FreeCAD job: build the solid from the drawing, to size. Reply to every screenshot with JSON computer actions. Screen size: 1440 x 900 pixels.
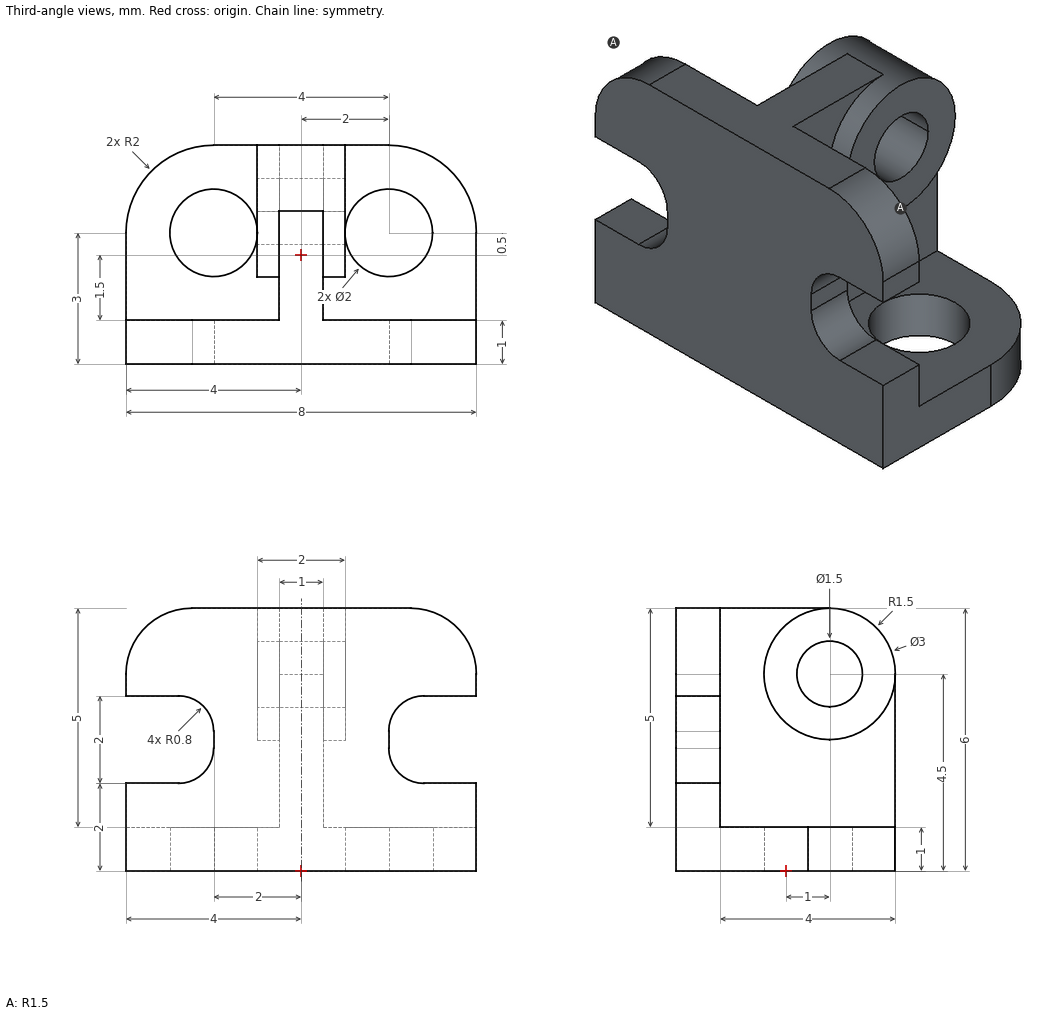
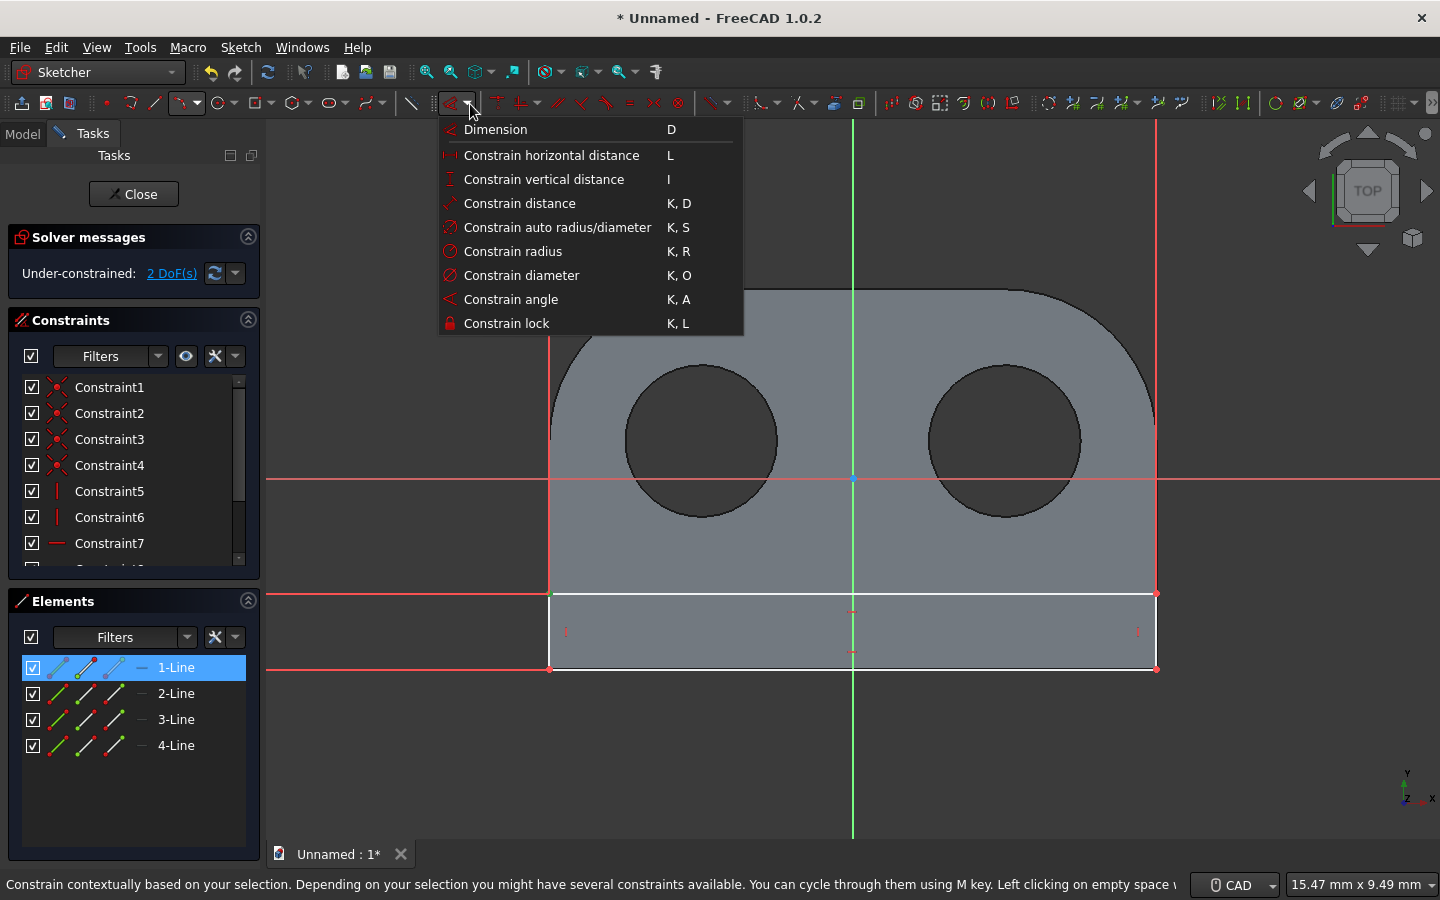
{"action": "left_click", "coordinate": [591, 155]}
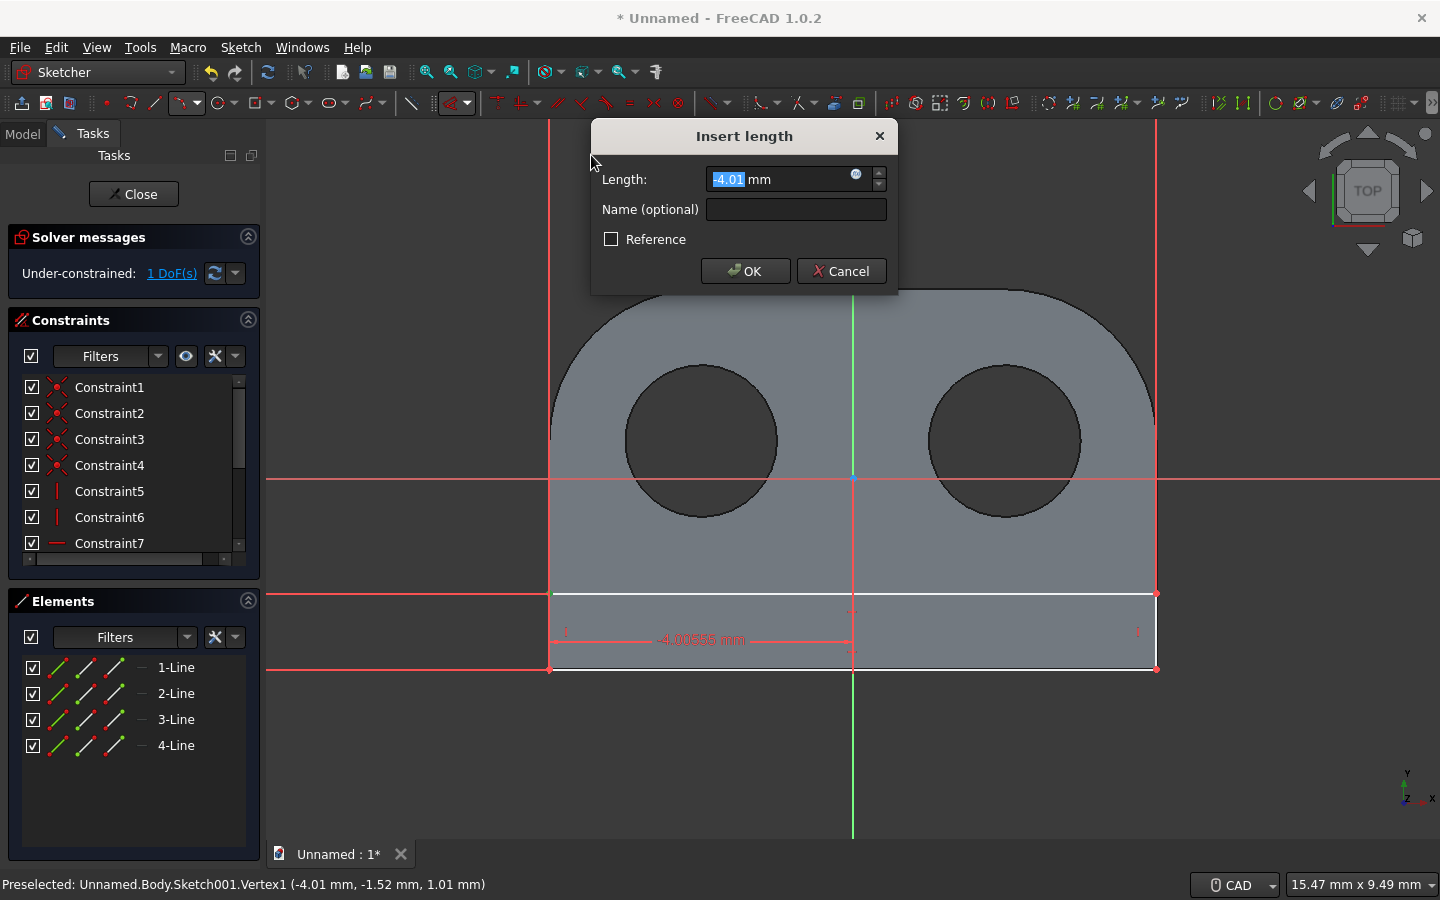
{"action": "type", "text": "-4"}
{"action": "key", "text": "Return"}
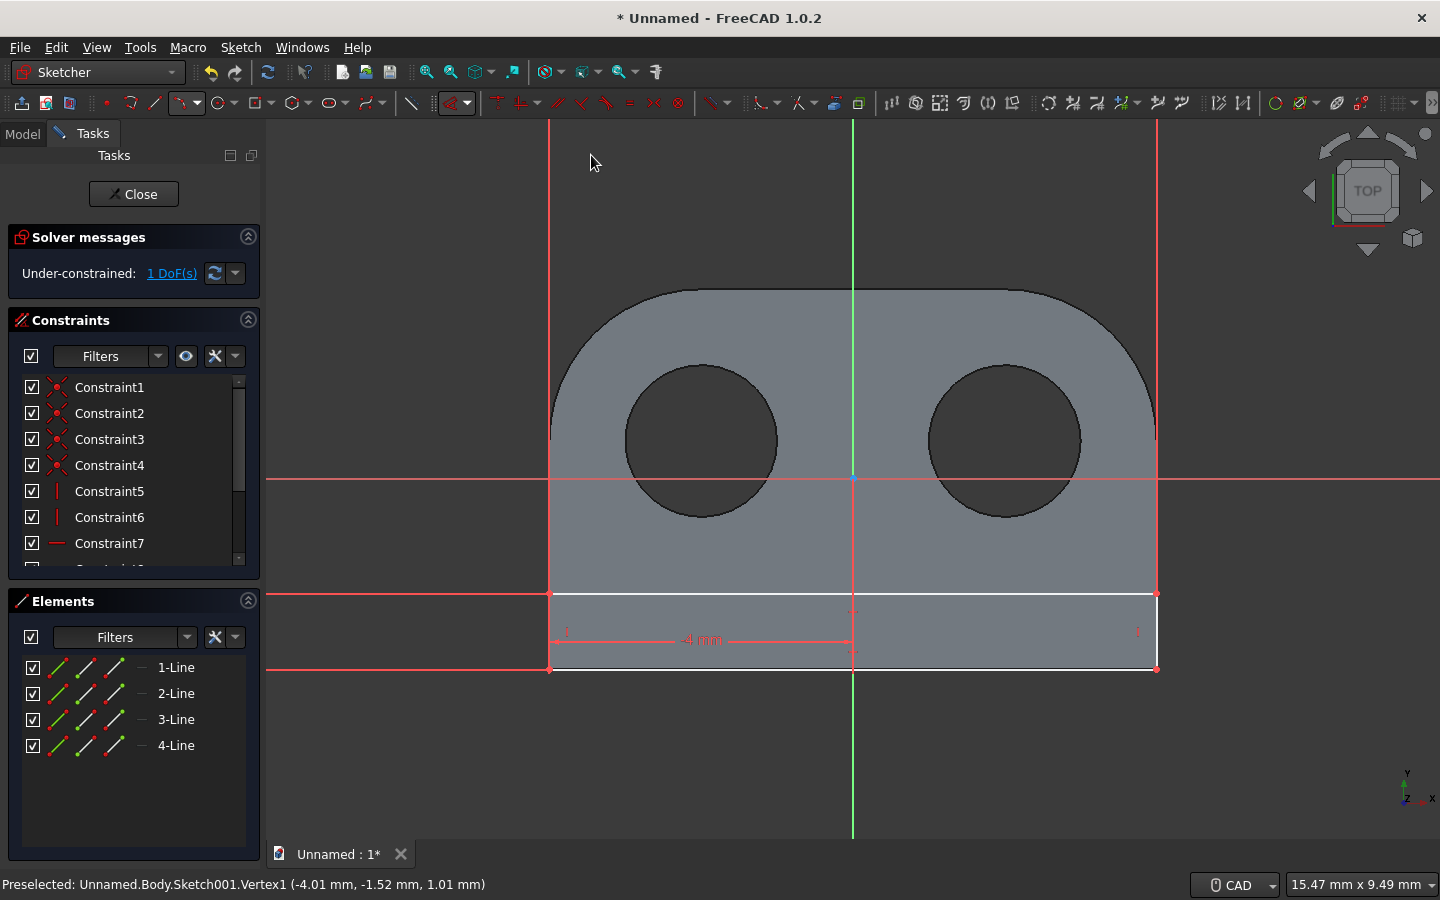
{"action": "left_click", "coordinate": [549, 594]}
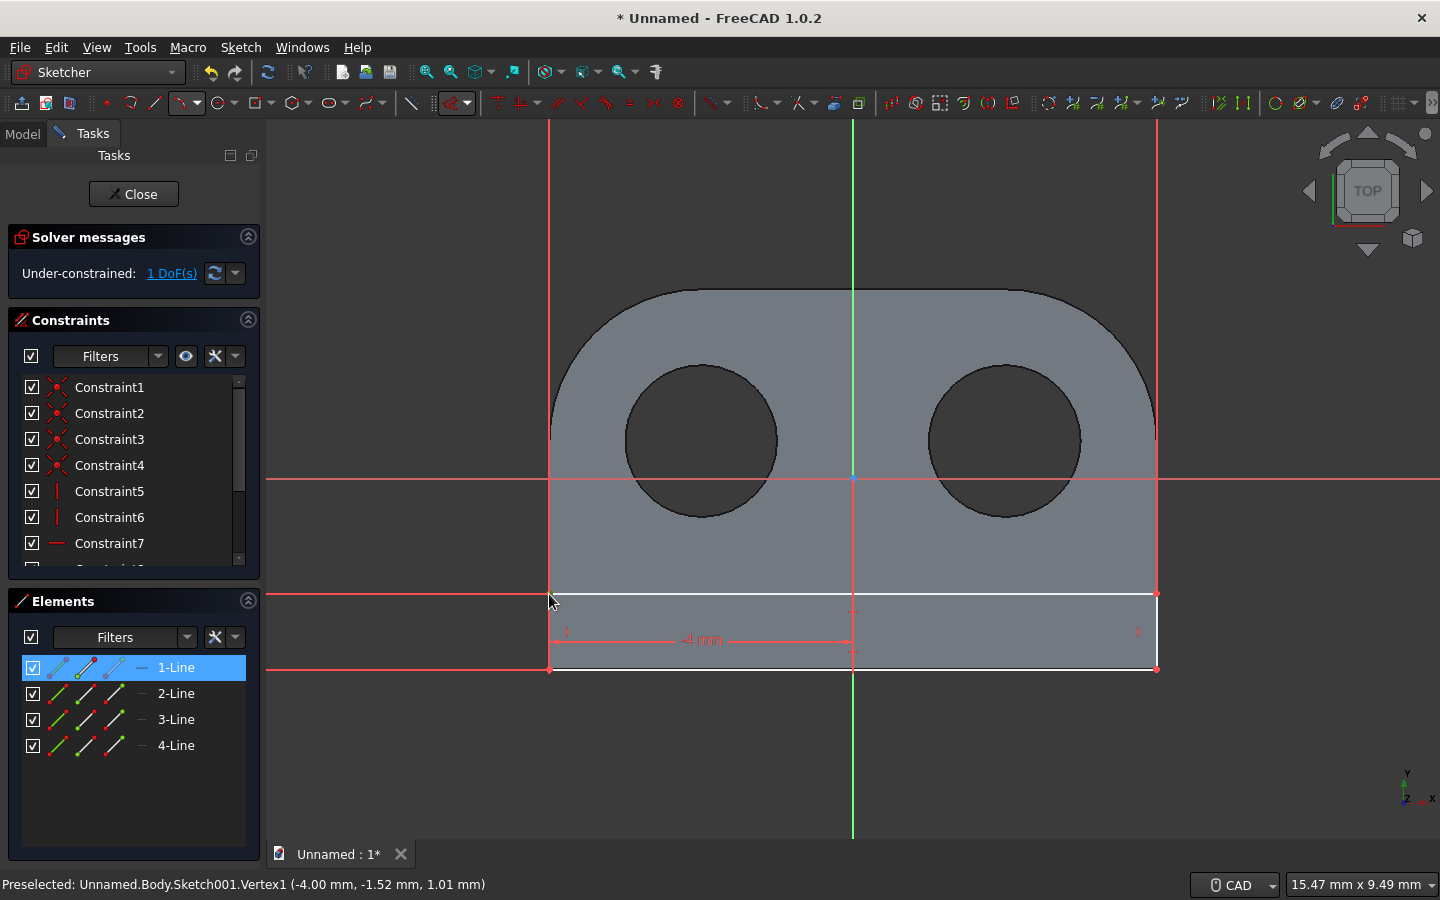
{"action": "key", "text": "i"}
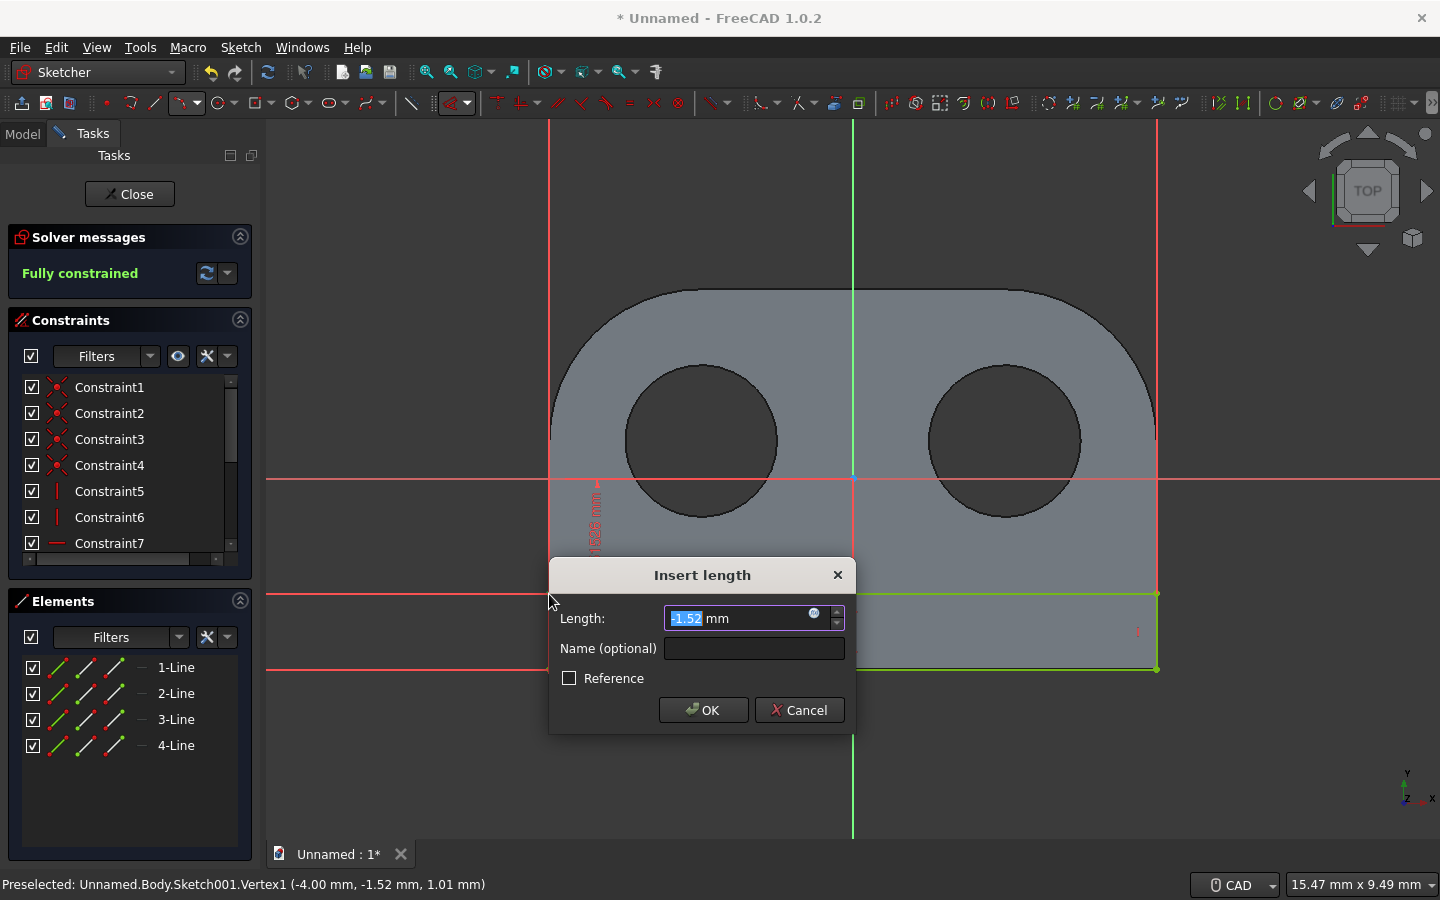
{"action": "type", "text": "-1.5"}
{"action": "key", "text": "Return"}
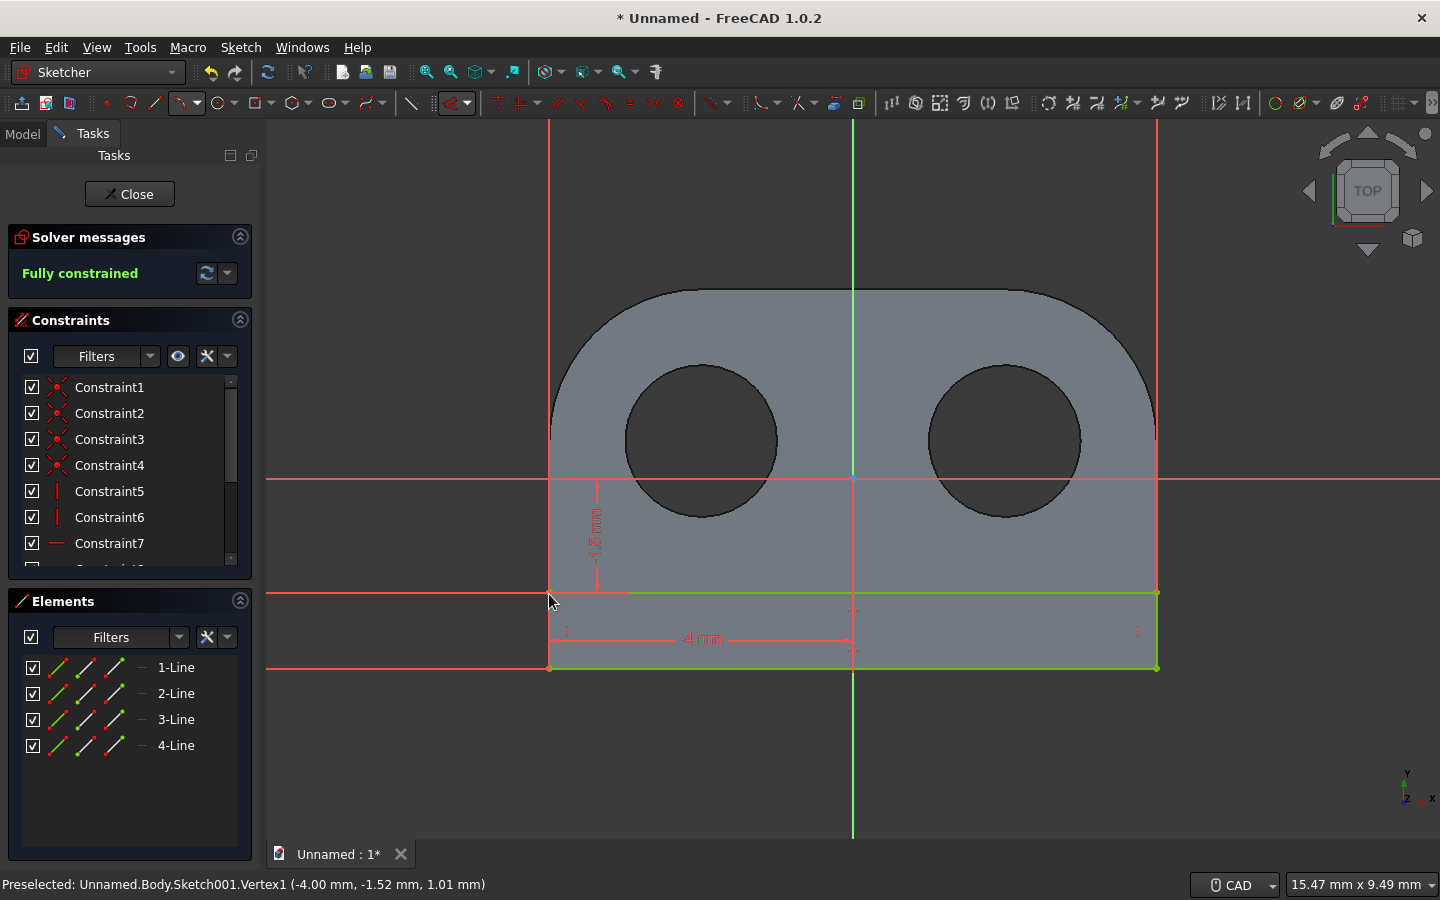
{"action": "left_click", "coordinate": [130, 194]}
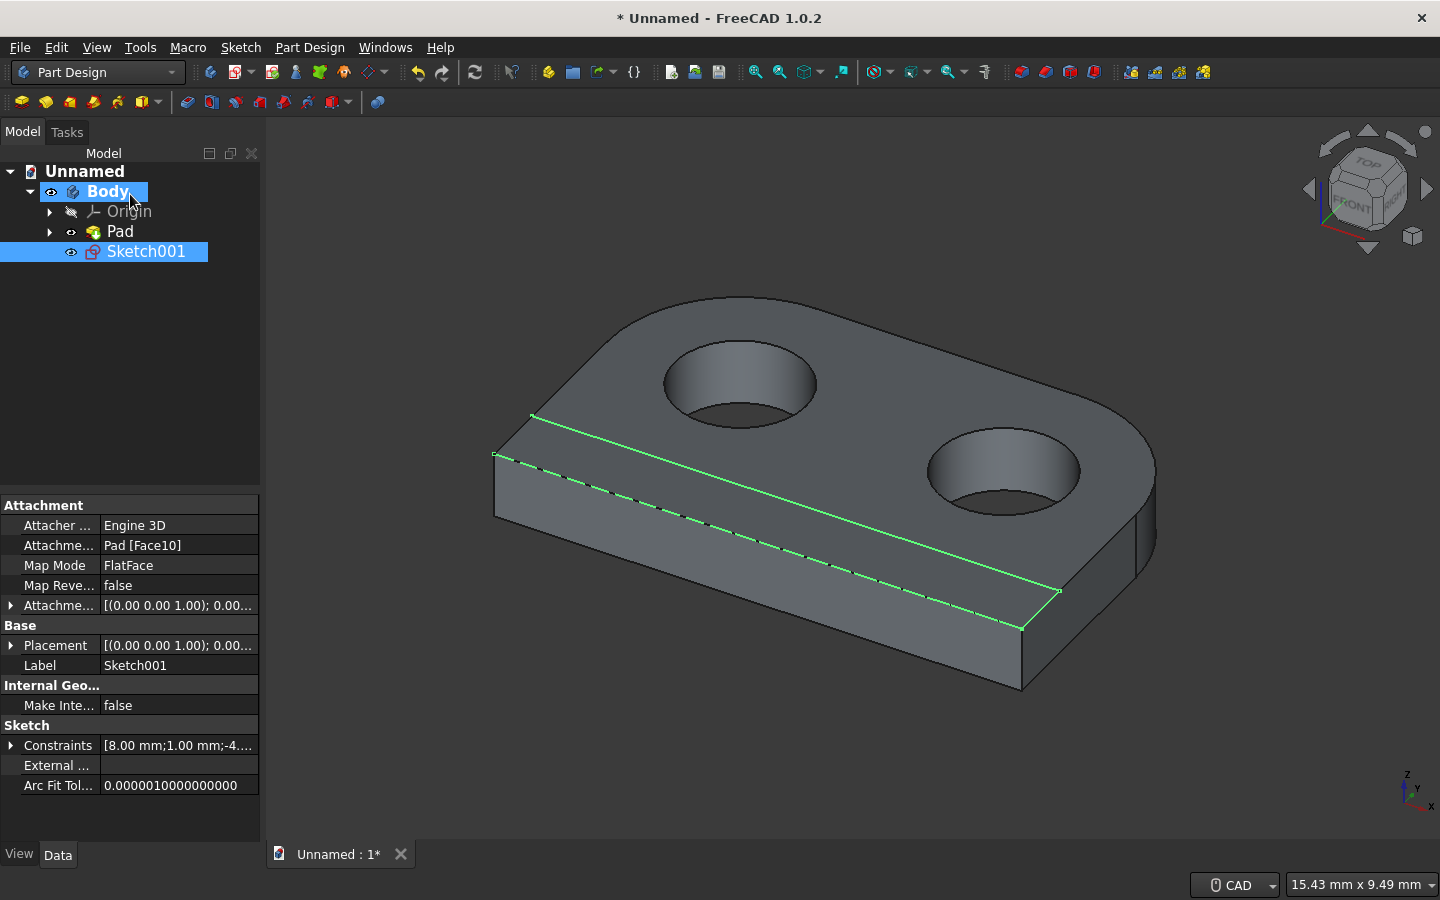
{"action": "left_click", "coordinate": [22, 102]}